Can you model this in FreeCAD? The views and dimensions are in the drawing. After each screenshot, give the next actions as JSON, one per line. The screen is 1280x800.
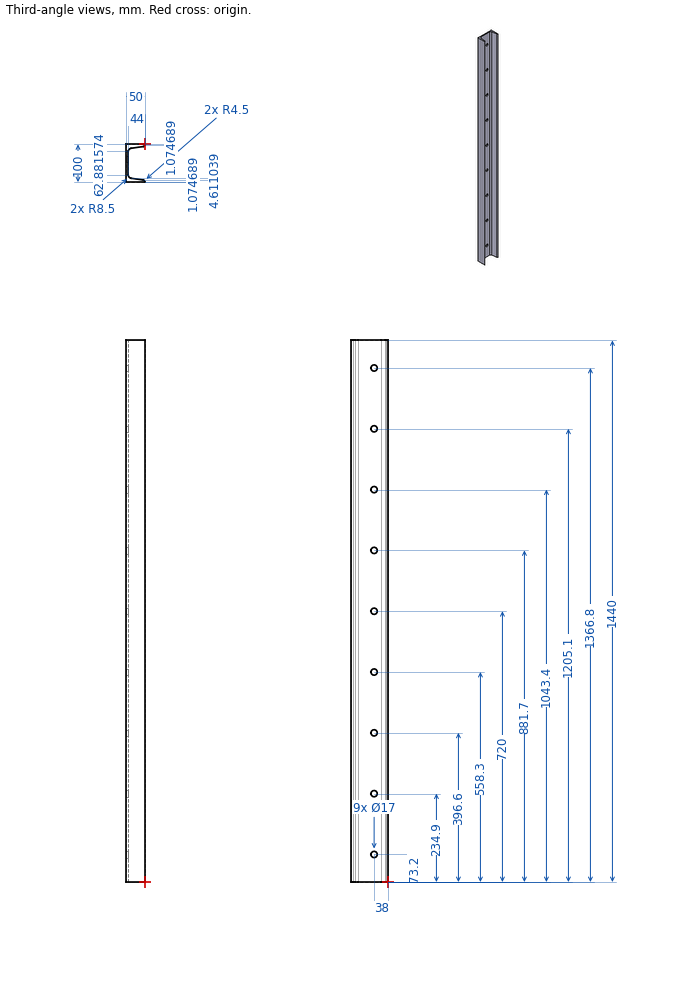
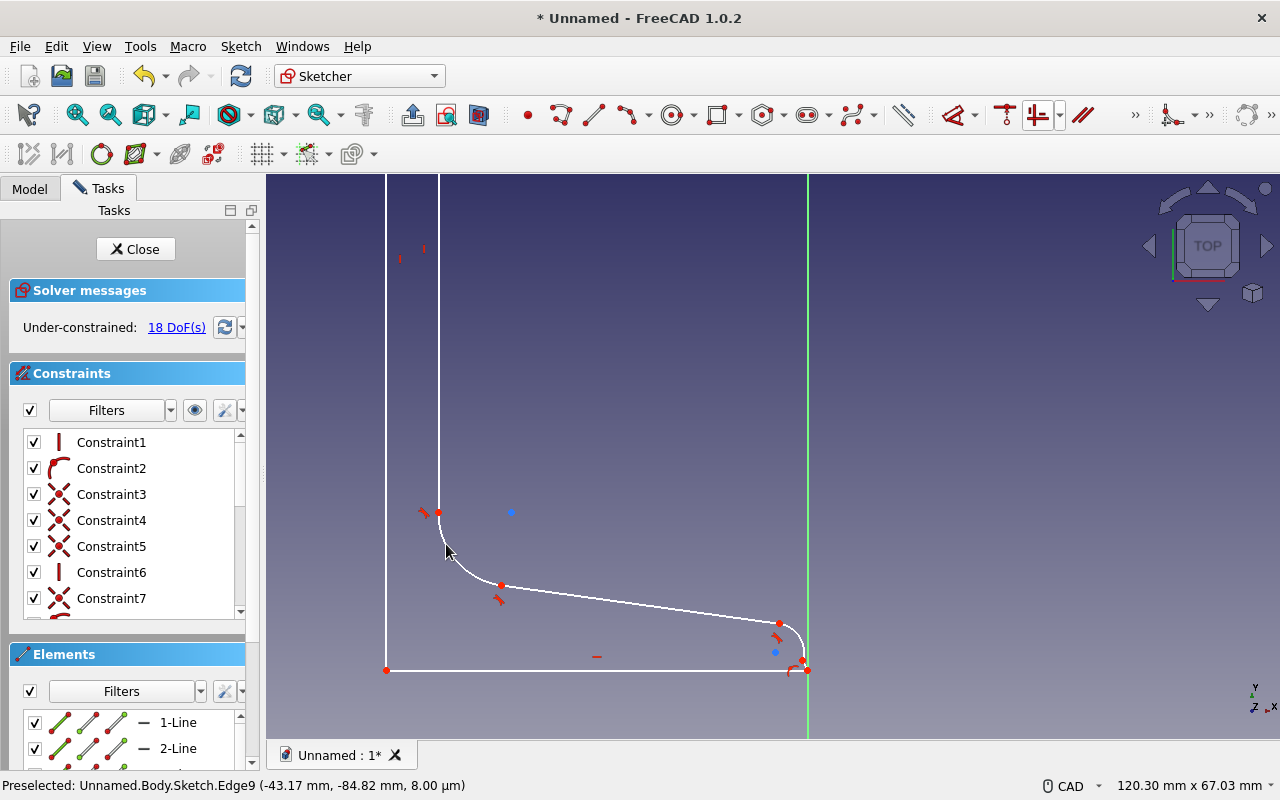
{"action": "left_click", "coordinate": [439, 354]}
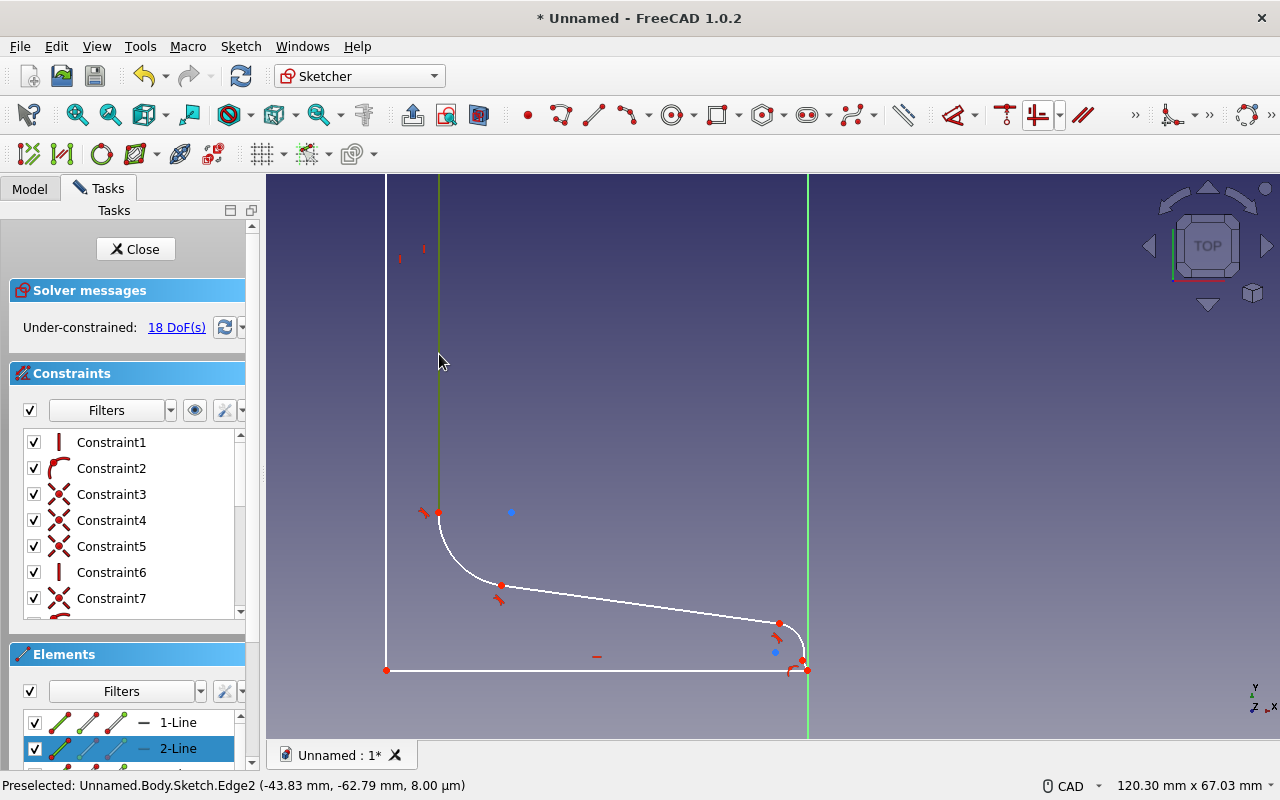
{"action": "scroll", "coordinate": [792, 627], "scroll_direction": "down", "scroll_amount": 4}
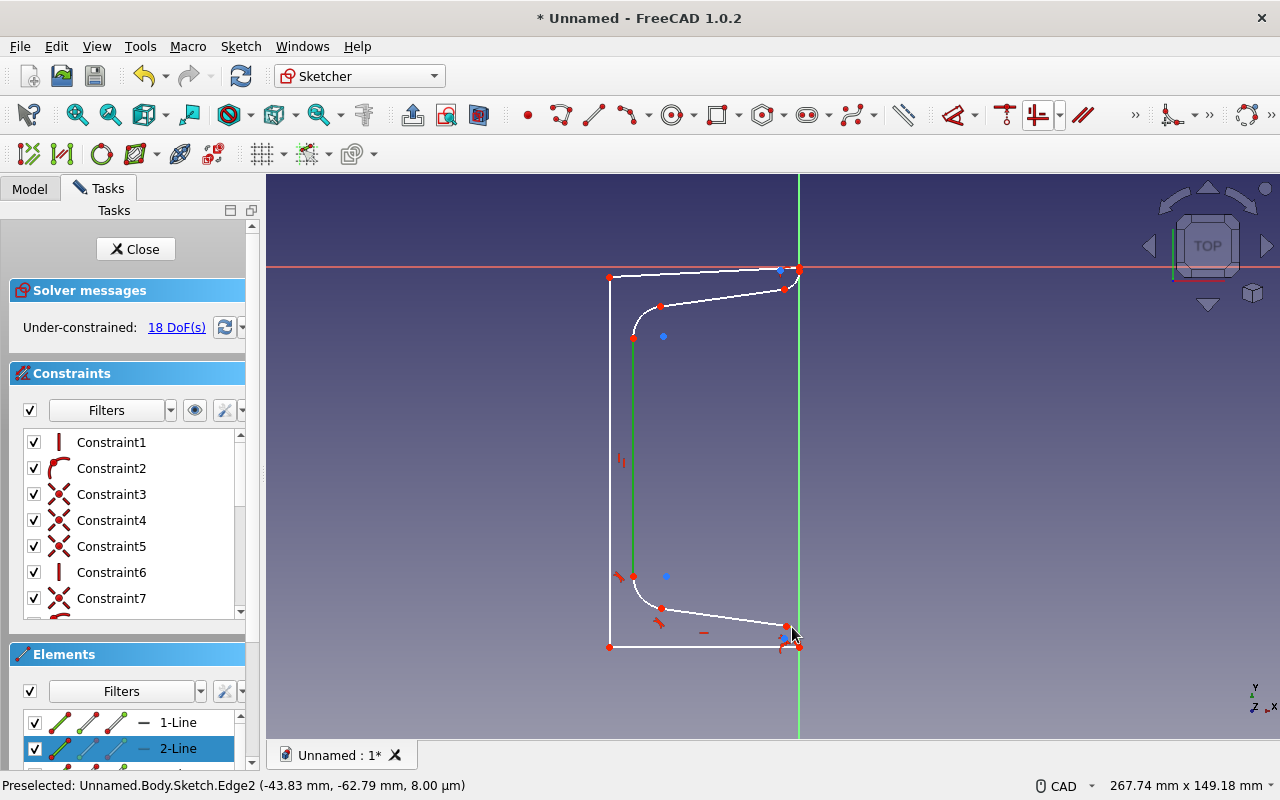
{"action": "left_click", "coordinate": [647, 311]}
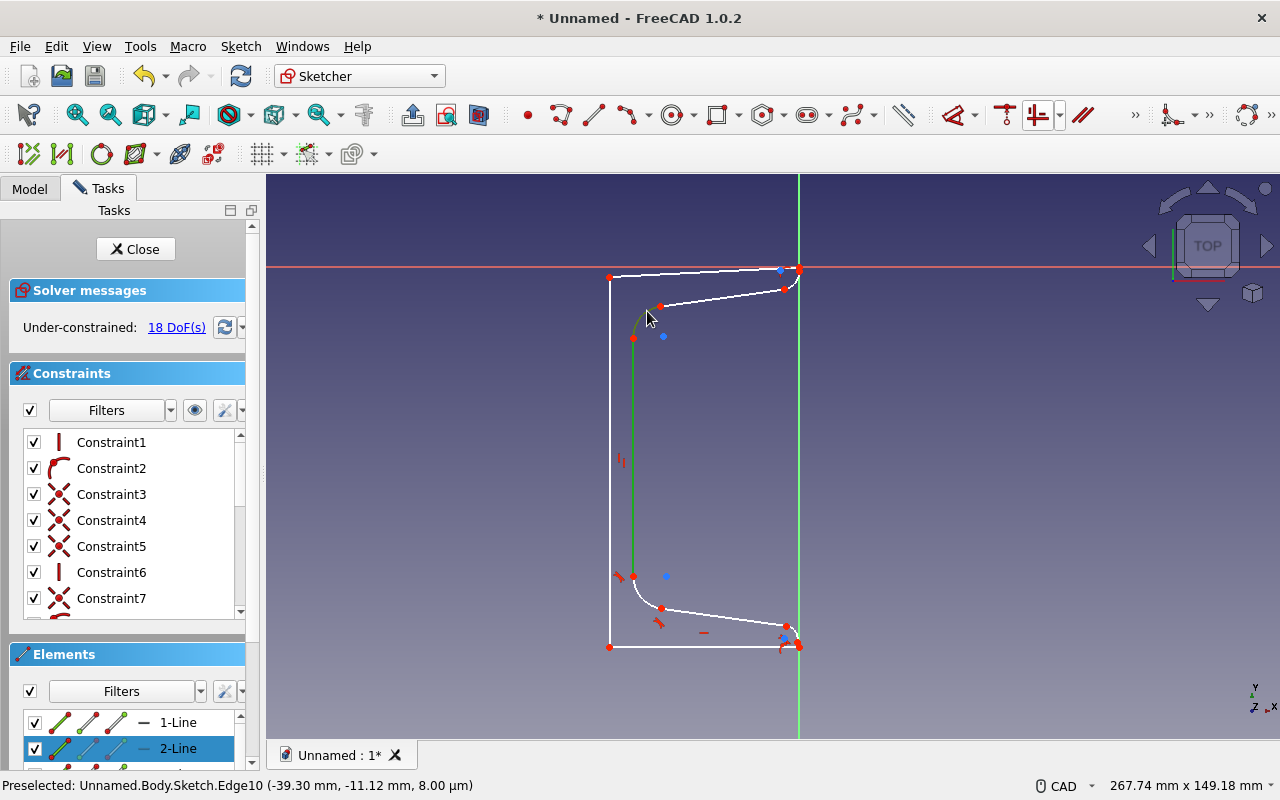
{"action": "key", "text": "t"}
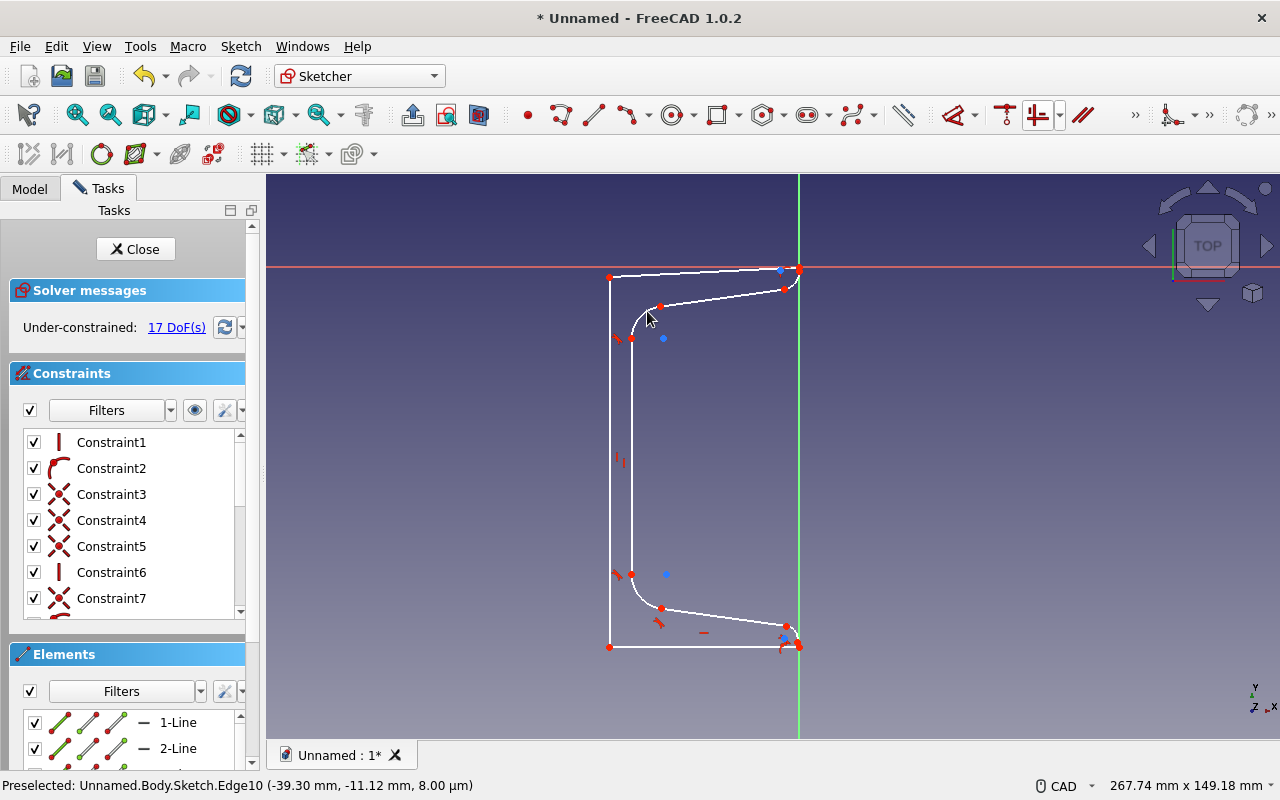
{"action": "left_click", "coordinate": [698, 302]}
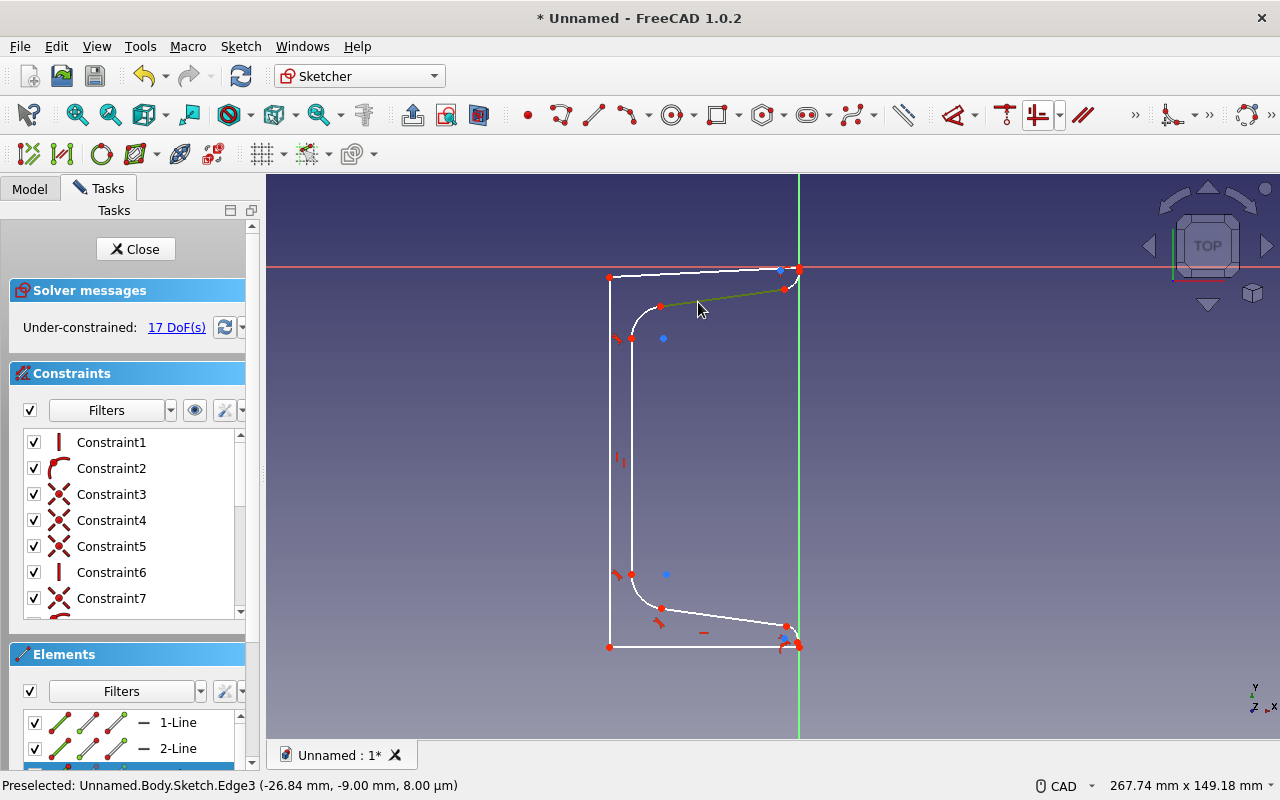
{"action": "left_click", "coordinate": [647, 311]}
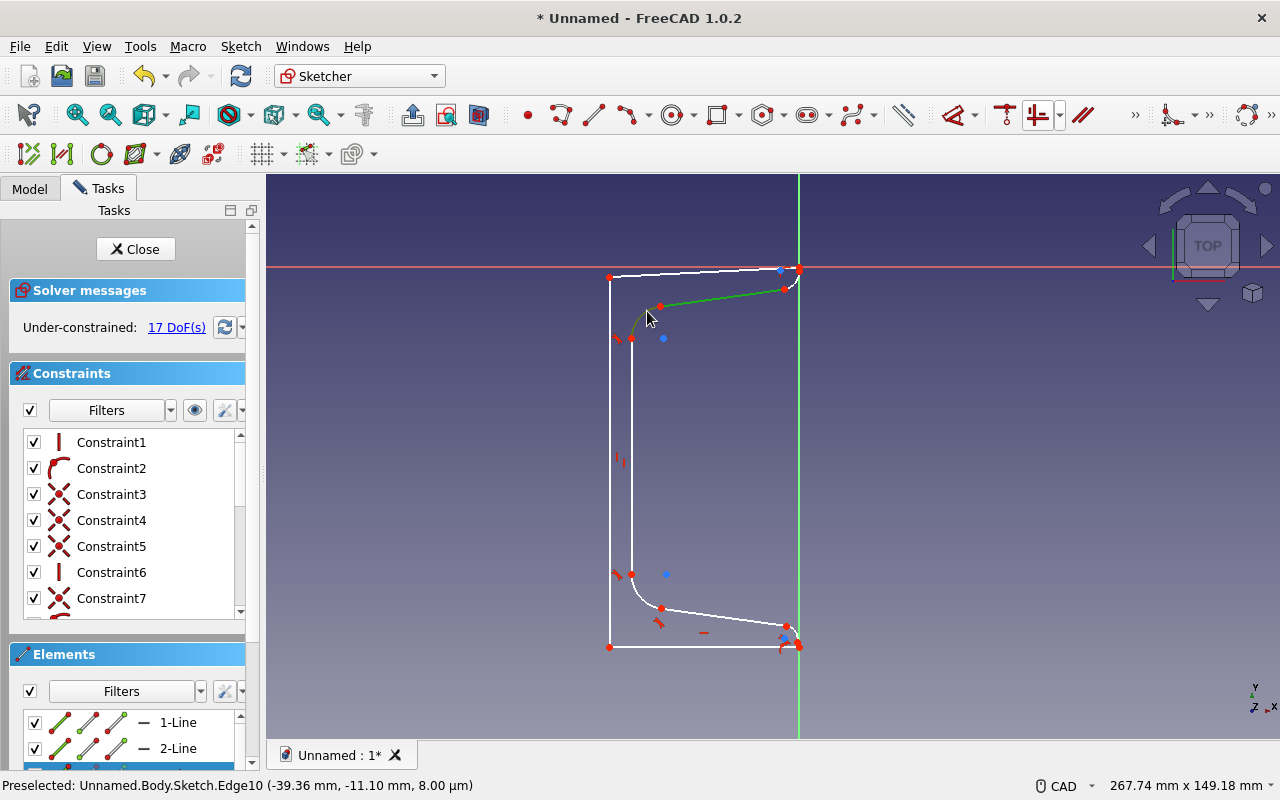
{"action": "key", "text": "t"}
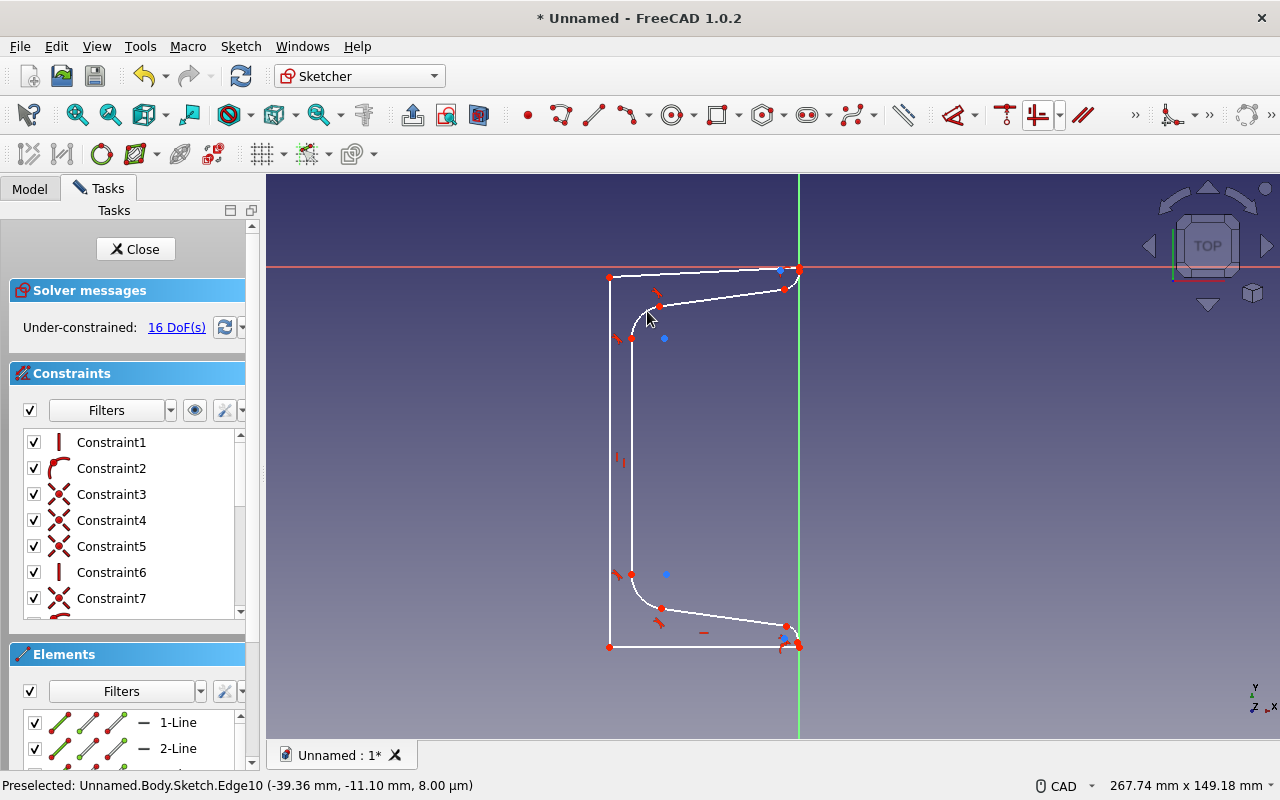
{"action": "left_click", "coordinate": [697, 301]}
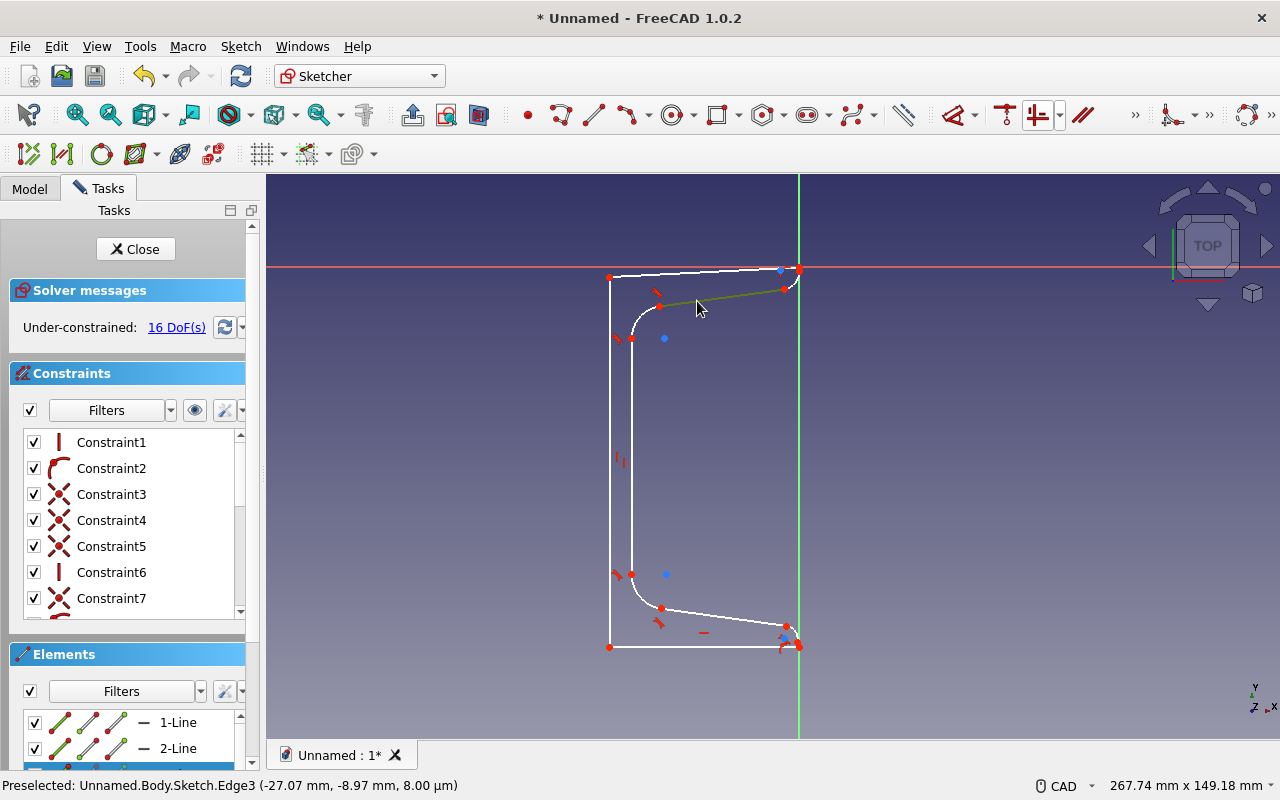
{"action": "scroll", "coordinate": [791, 286], "scroll_direction": "up", "scroll_amount": 4}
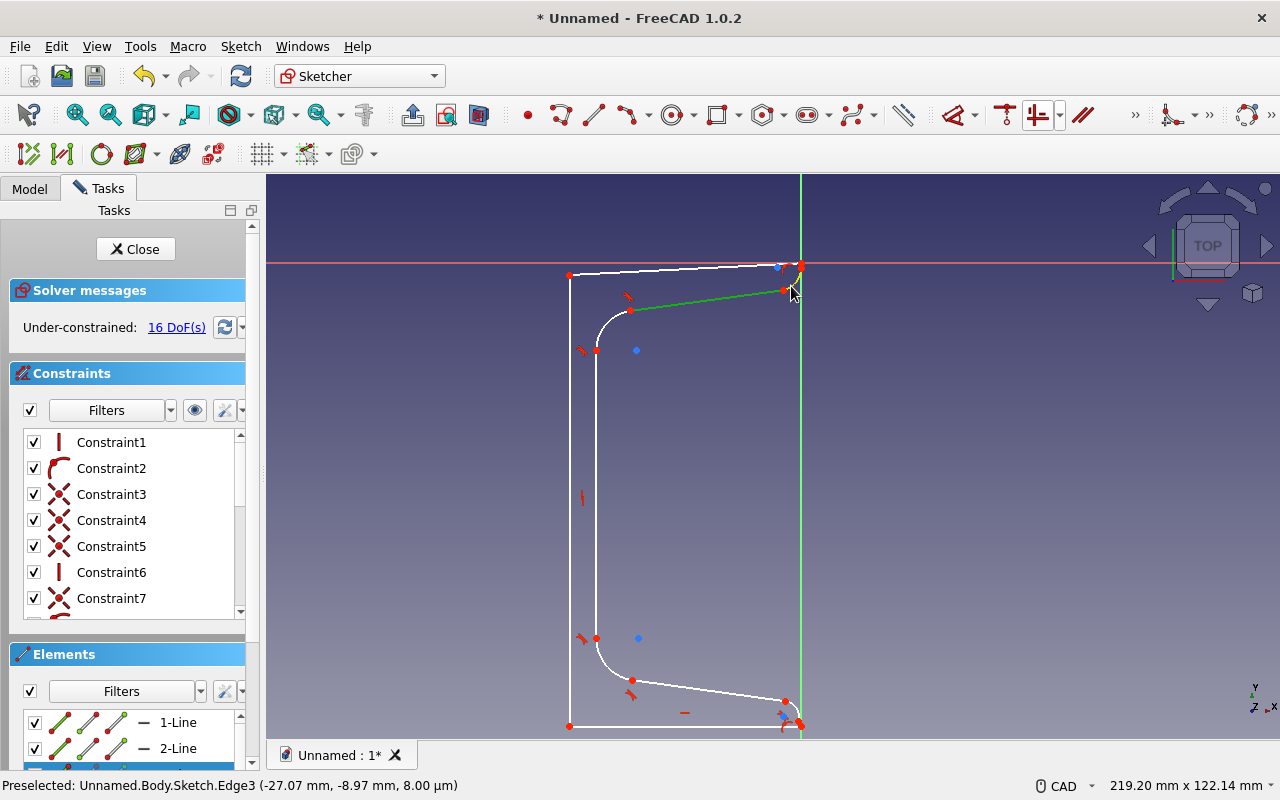
{"action": "left_click", "coordinate": [791, 287]}